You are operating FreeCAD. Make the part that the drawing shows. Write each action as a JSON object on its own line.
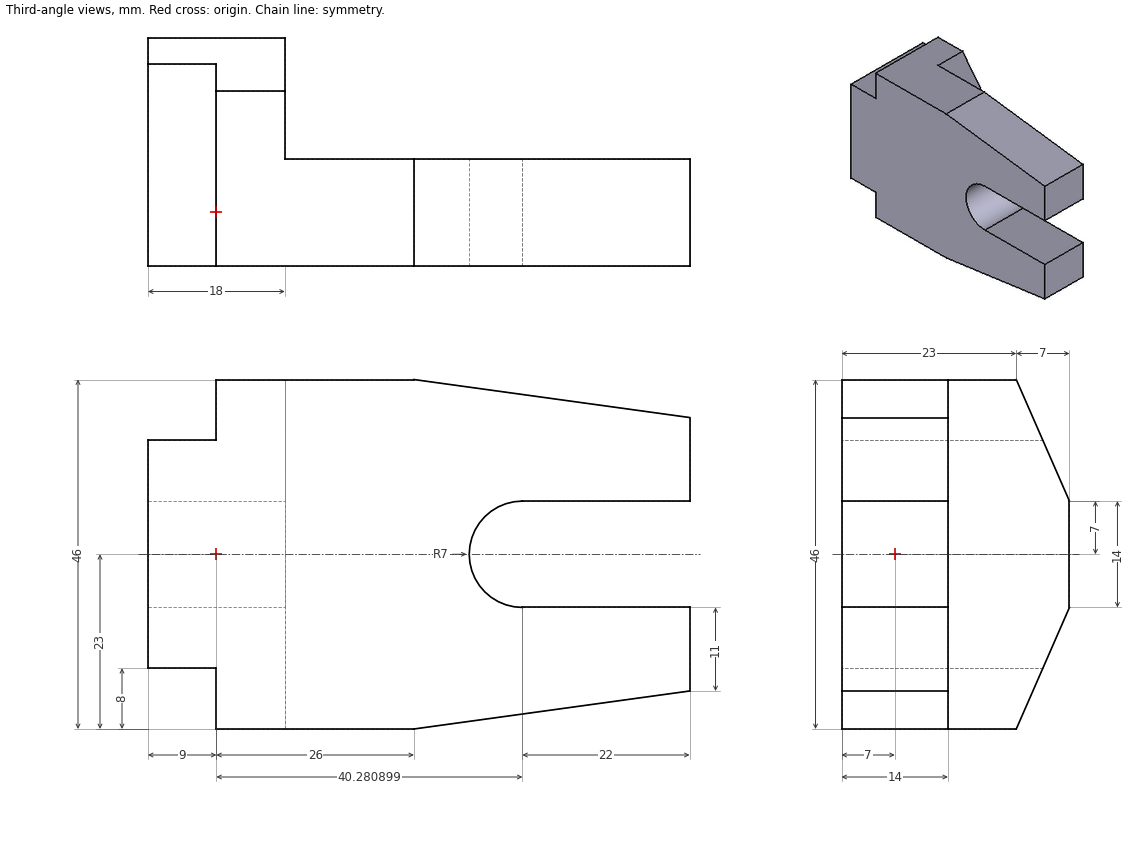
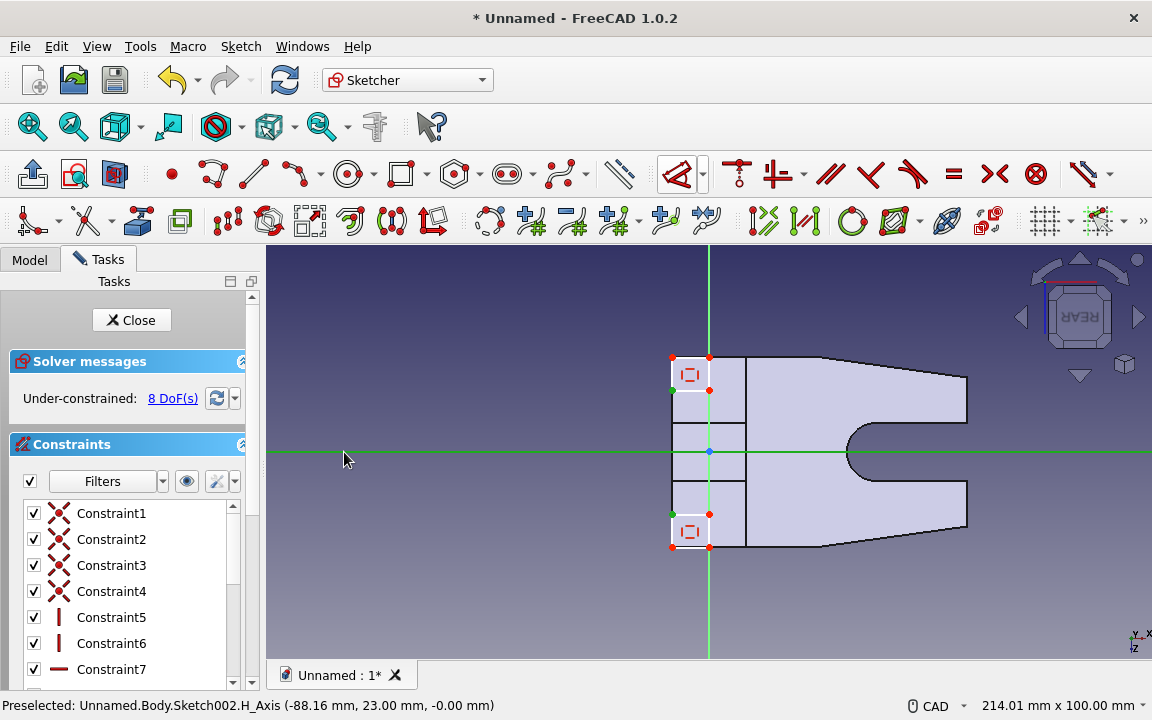
{"action": "key", "text": "s"}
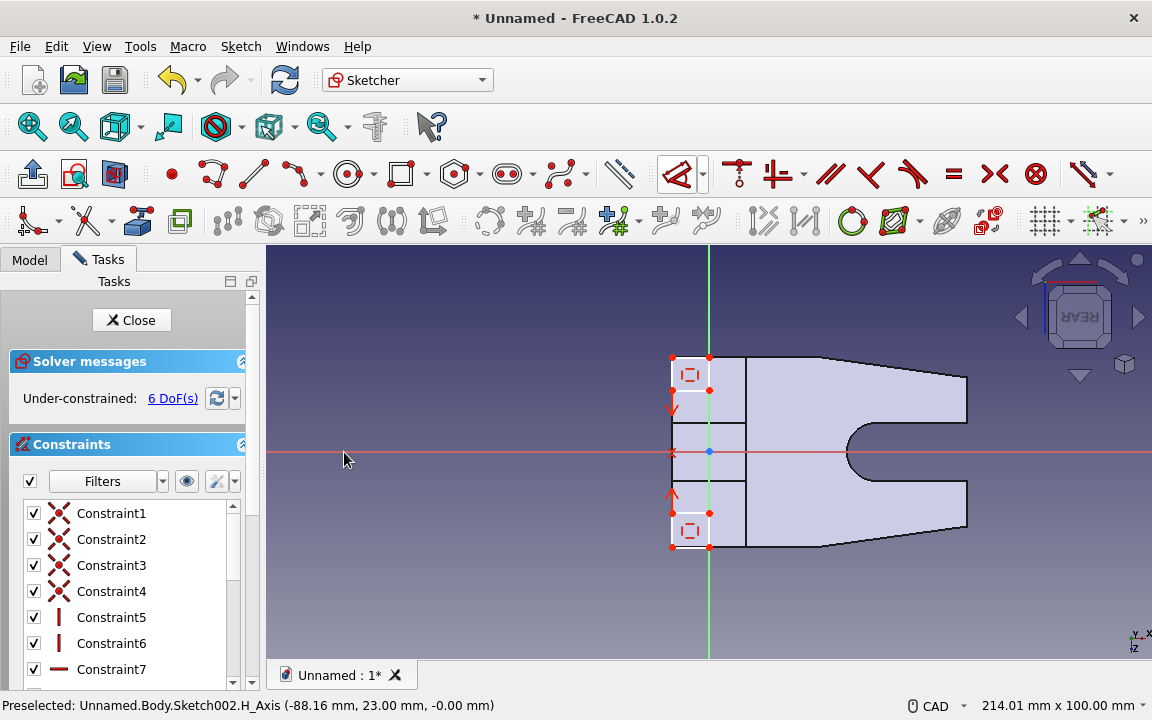
{"action": "left_click", "coordinate": [709, 358]}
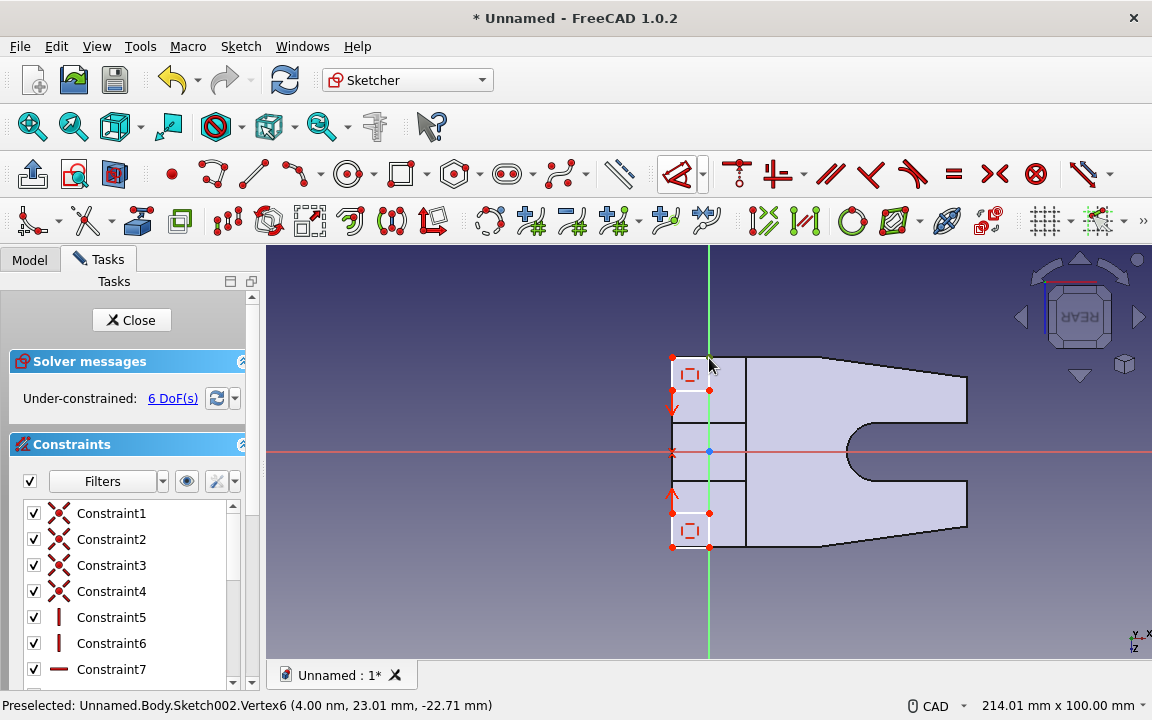
{"action": "left_click", "coordinate": [709, 548]}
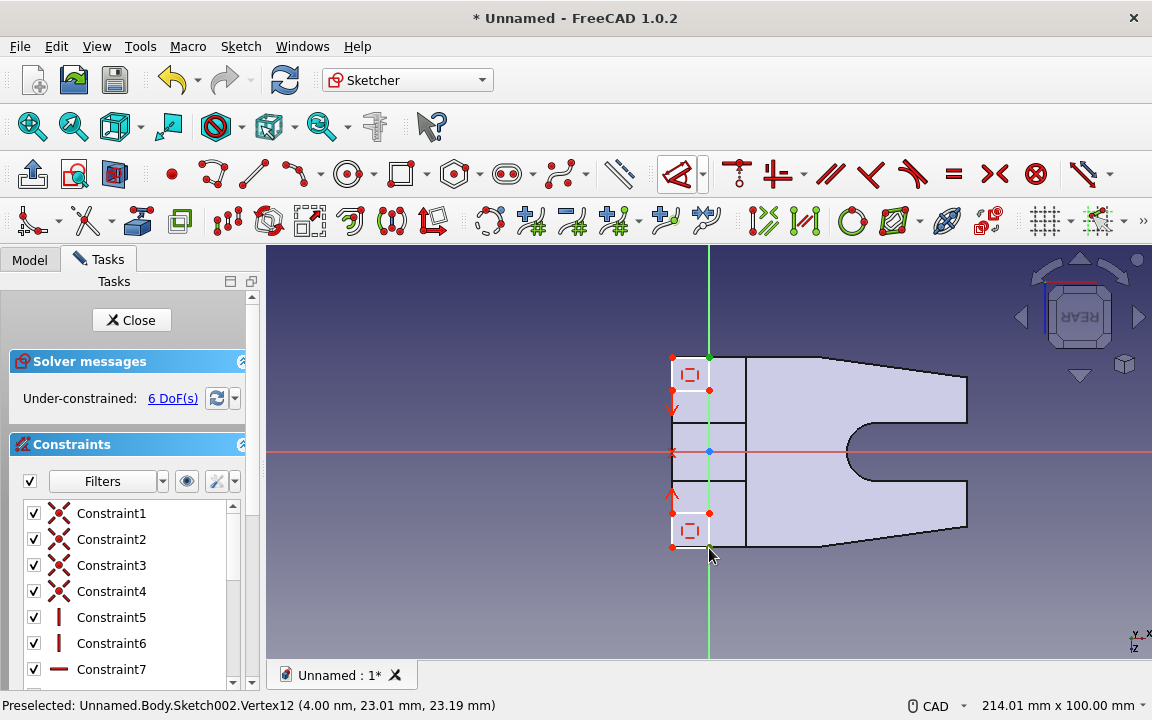
{"action": "left_click", "coordinate": [344, 452]}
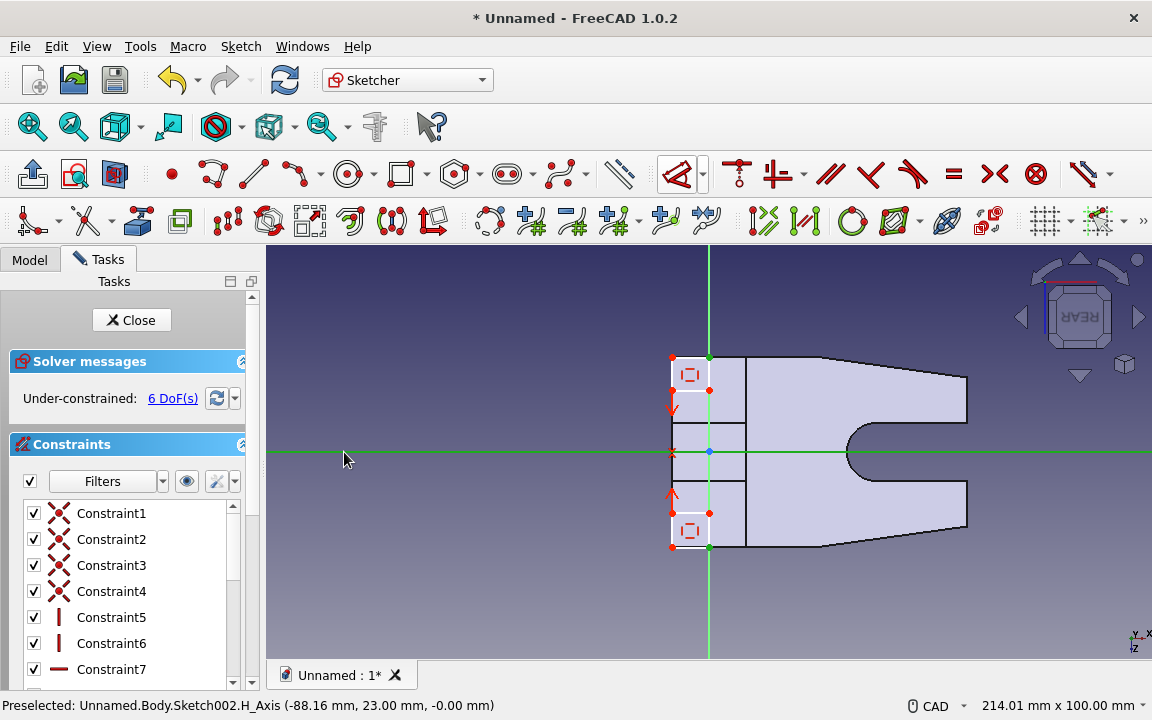
{"action": "key", "text": "s"}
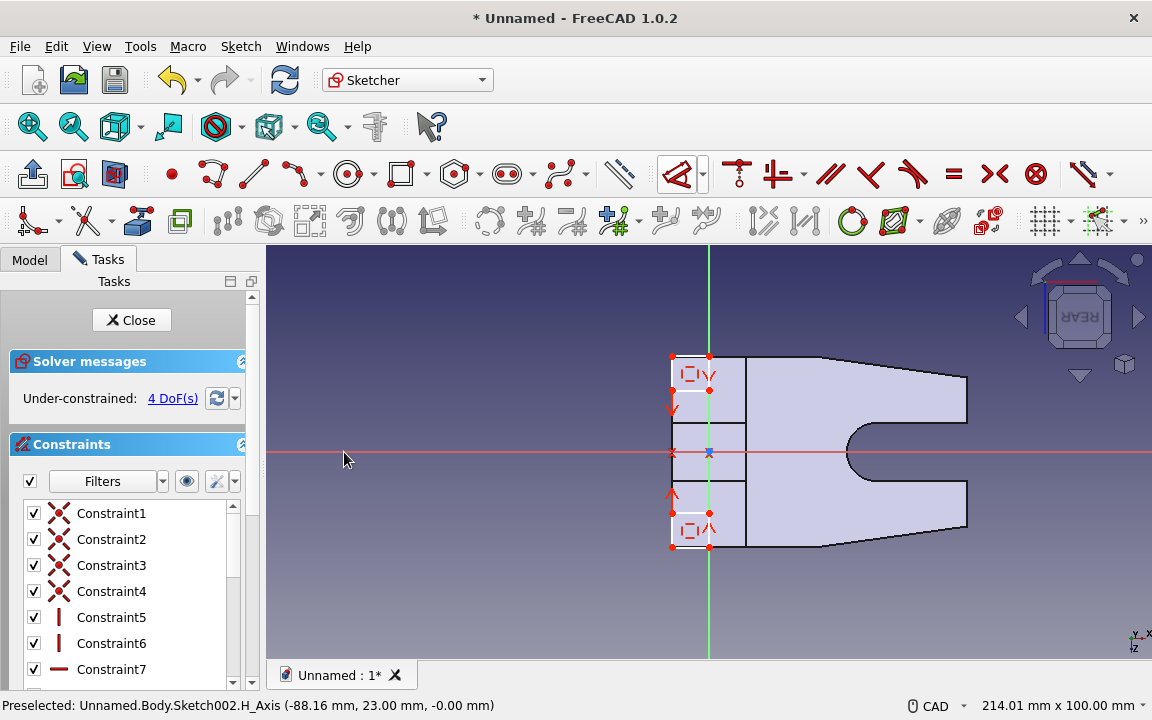
{"action": "left_click", "coordinate": [709, 391]}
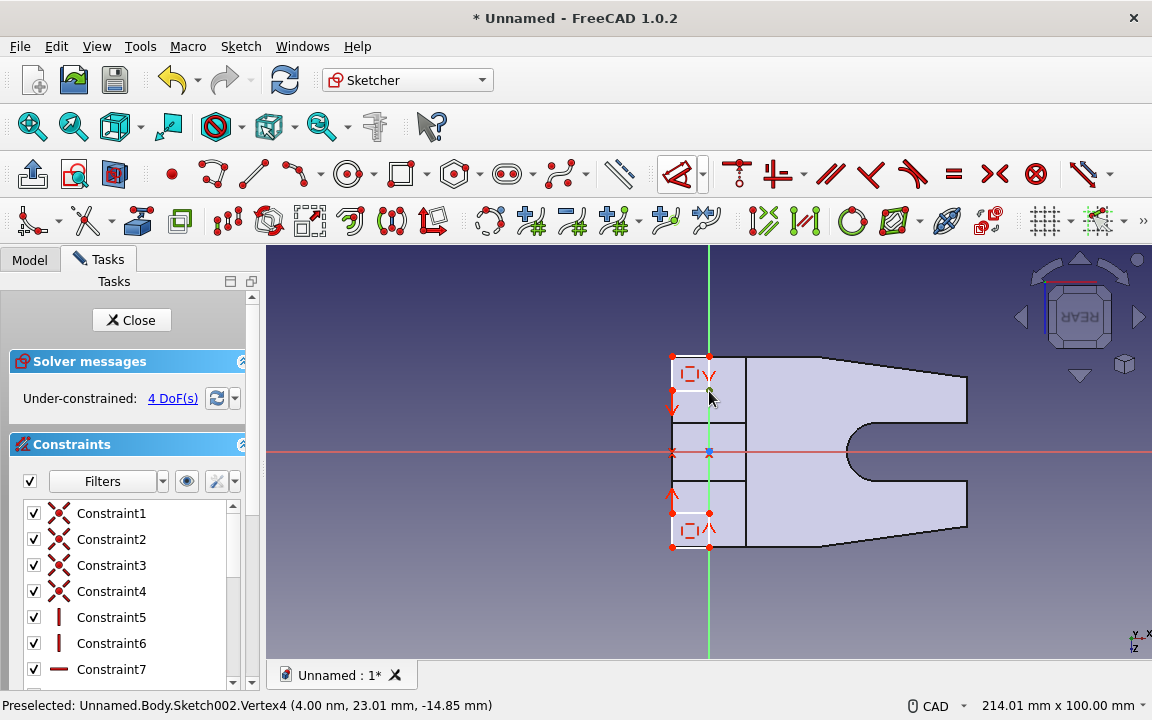
{"action": "left_click", "coordinate": [709, 605]}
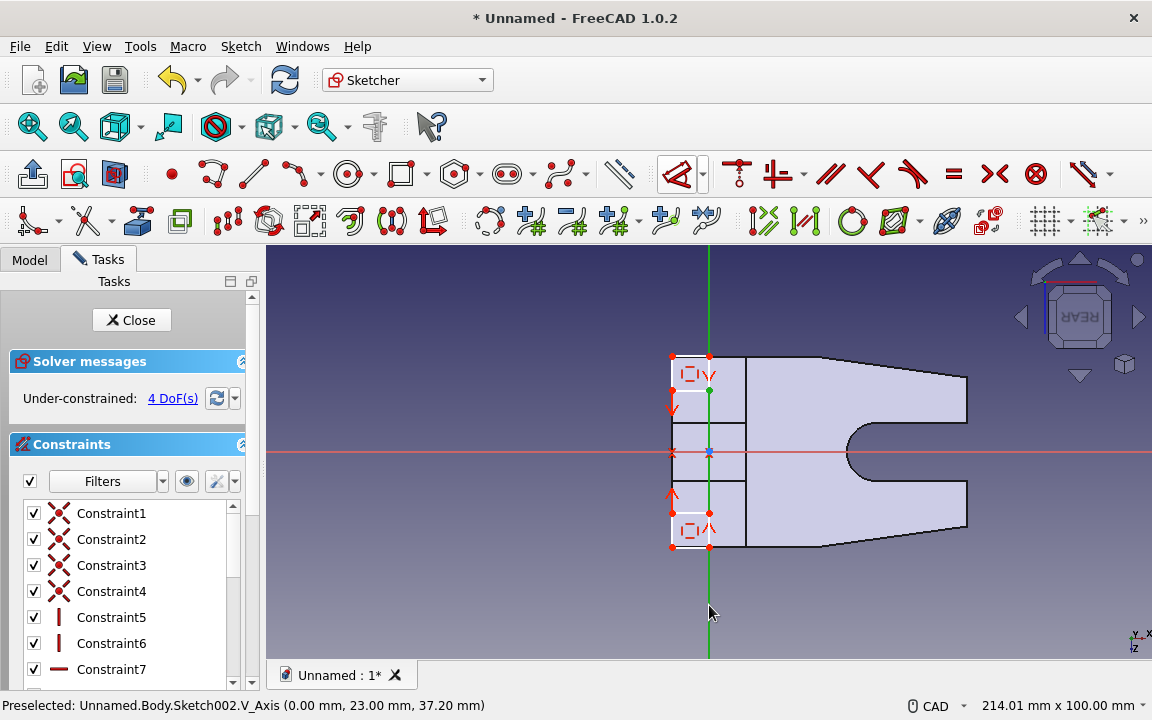
{"action": "left_click", "coordinate": [737, 174]}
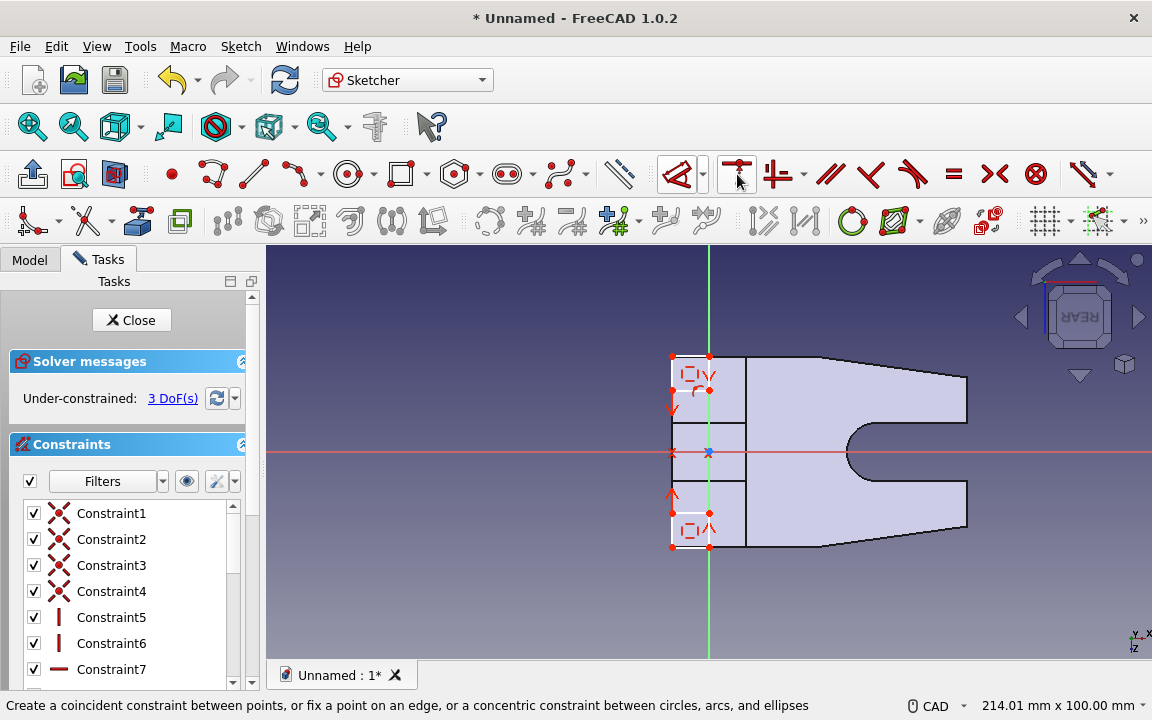
{"action": "scroll", "coordinate": [672, 367], "scroll_direction": "up", "scroll_amount": 2}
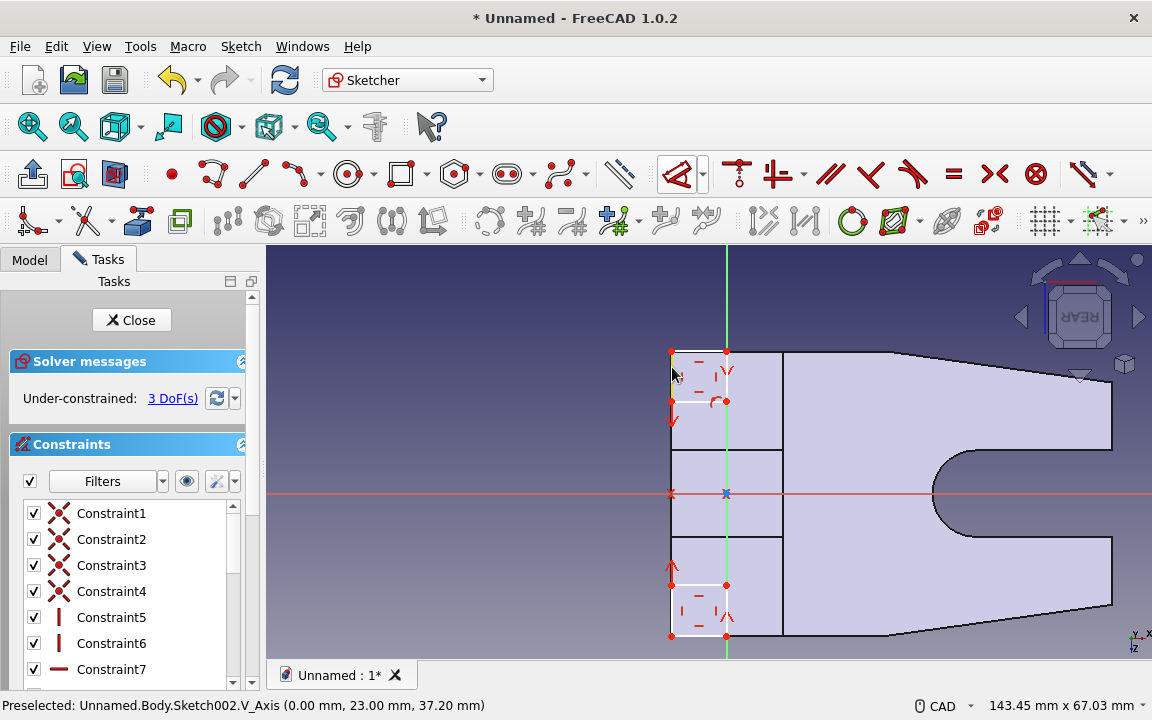
{"action": "left_click", "coordinate": [672, 366]}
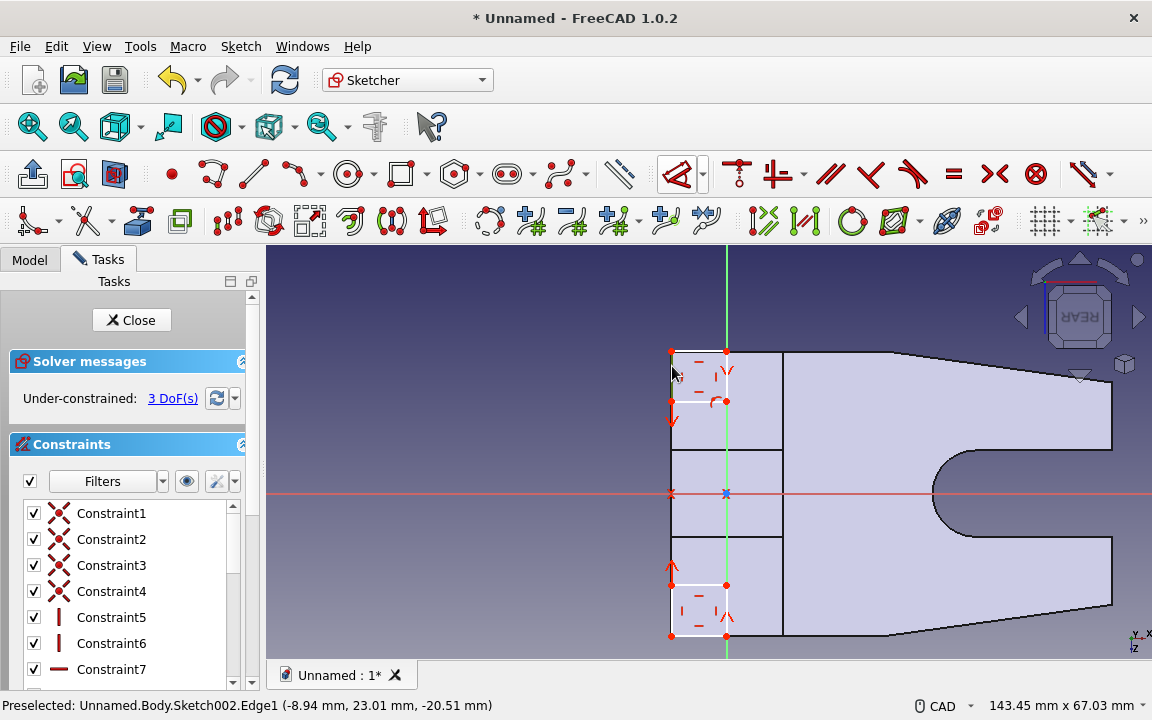
{"action": "key", "text": "i"}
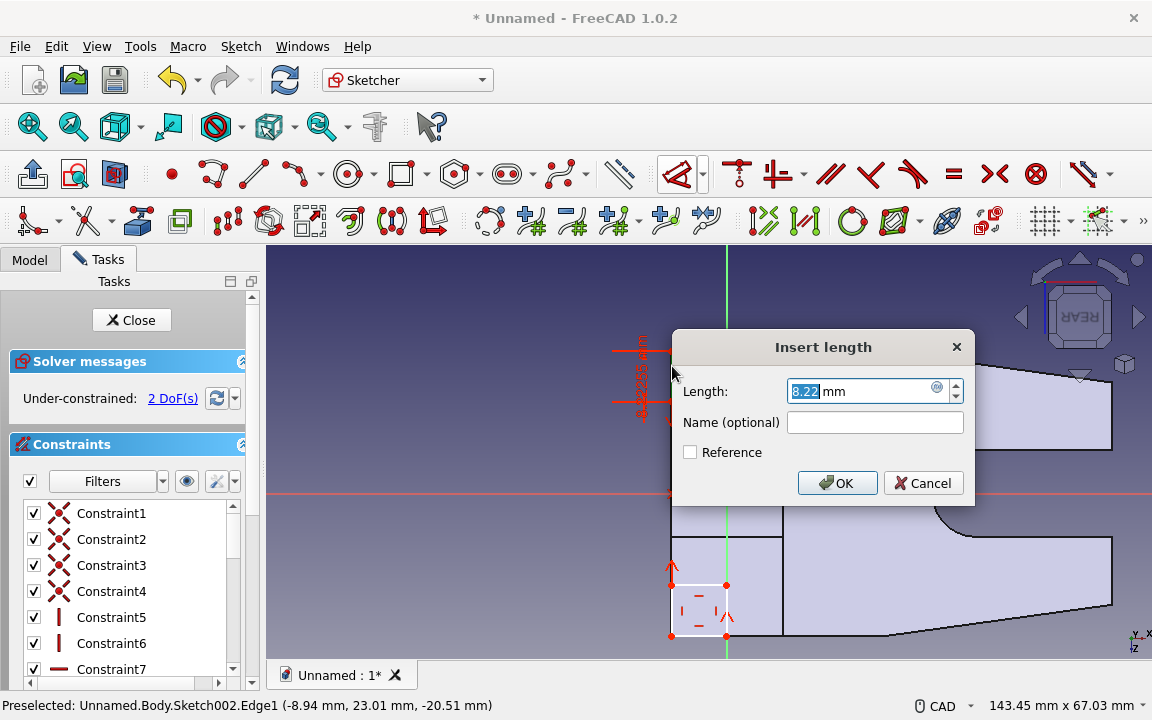
{"action": "type", "text": "8"}
{"action": "key", "text": "Return"}